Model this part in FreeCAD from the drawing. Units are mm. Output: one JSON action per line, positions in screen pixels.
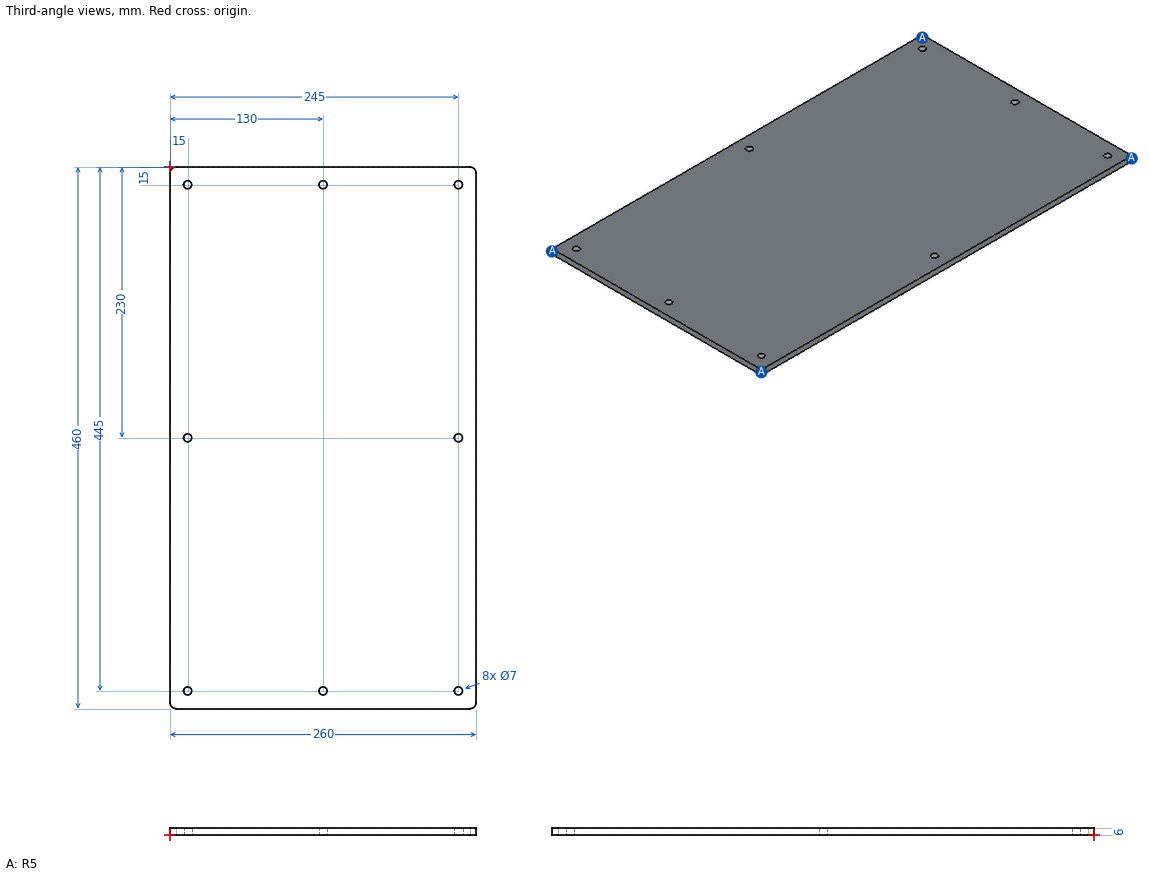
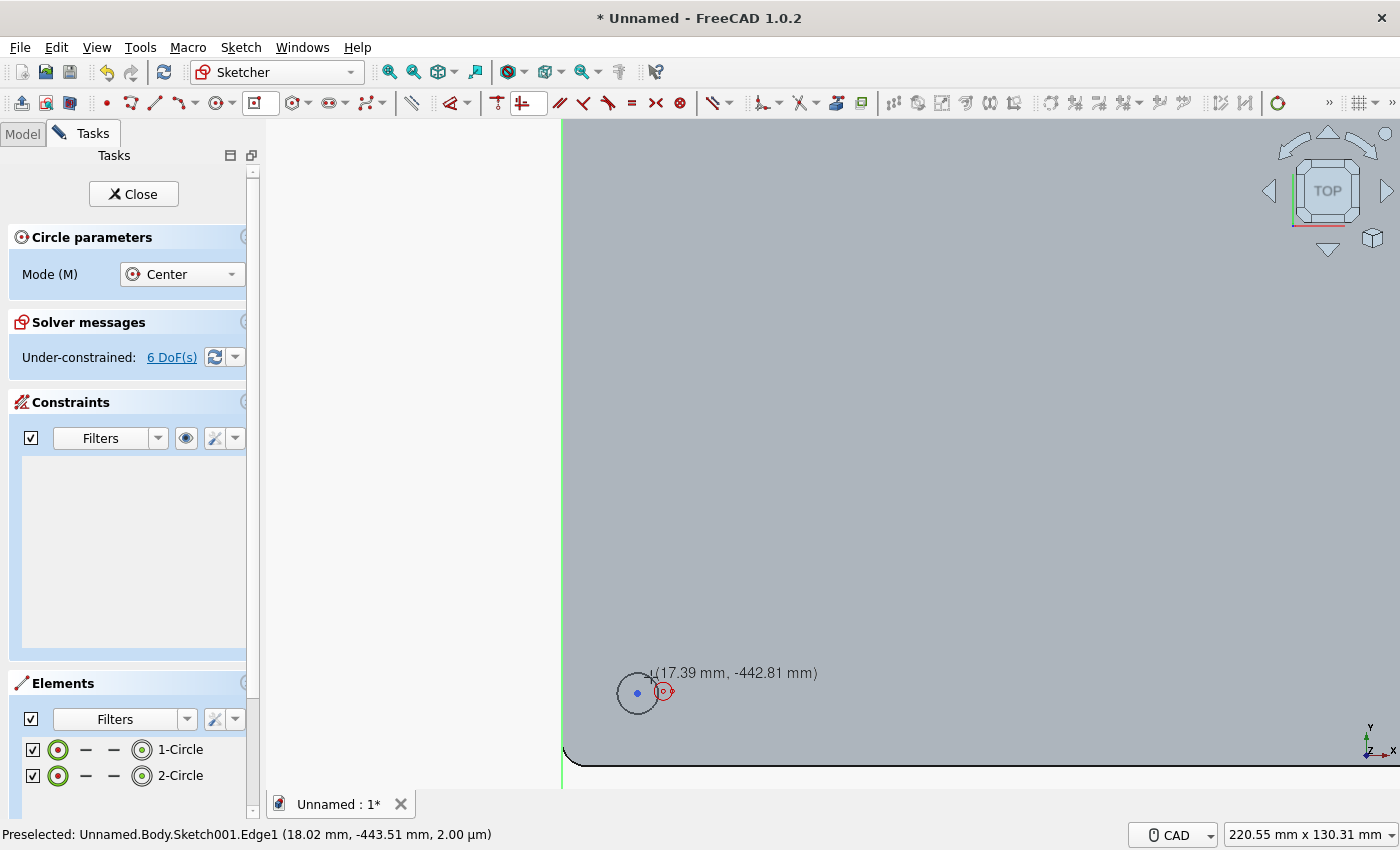
{"action": "scroll", "coordinate": [654, 682], "scroll_direction": "down", "scroll_amount": 8}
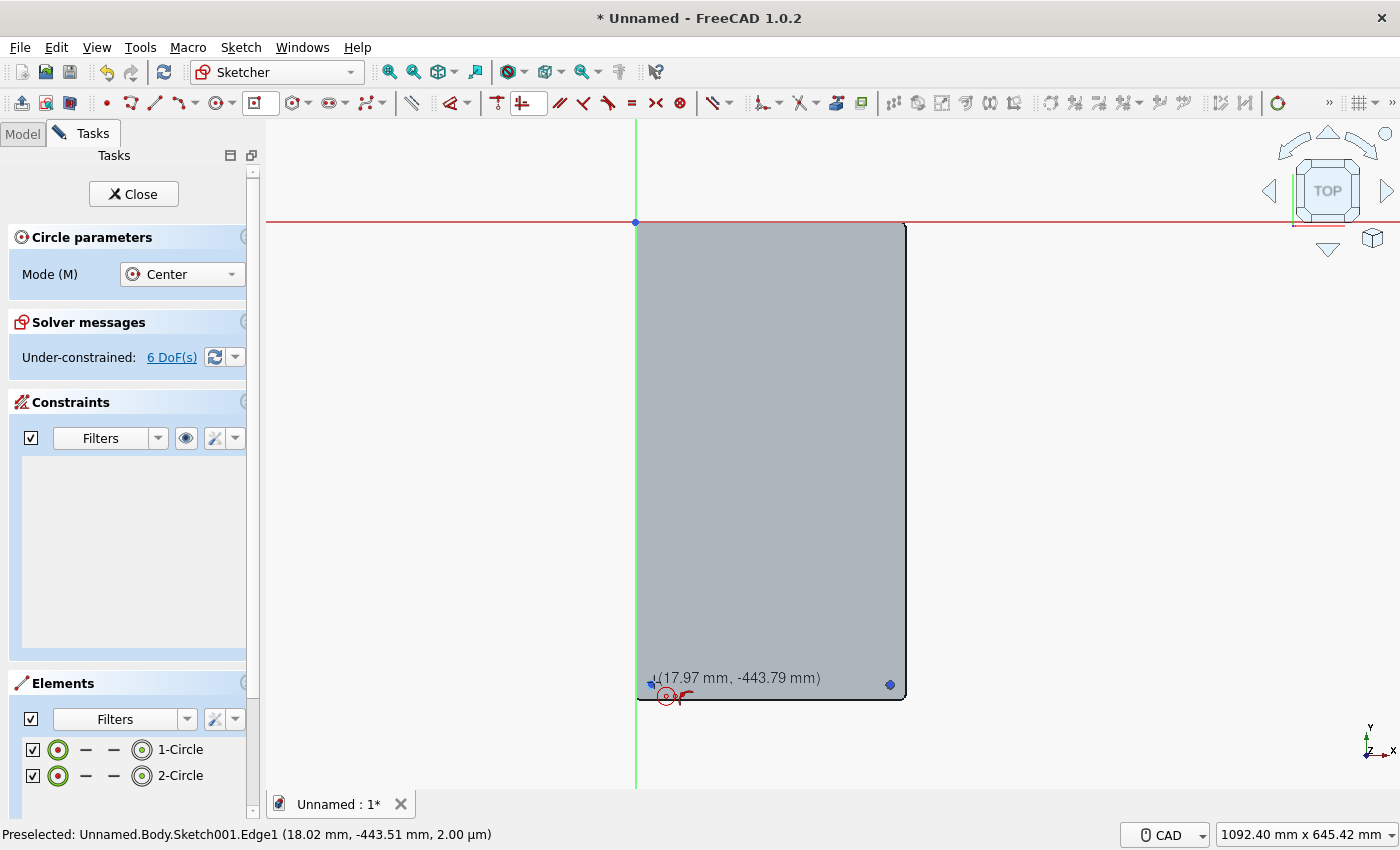
{"action": "scroll", "coordinate": [890, 238], "scroll_direction": "up", "scroll_amount": 10}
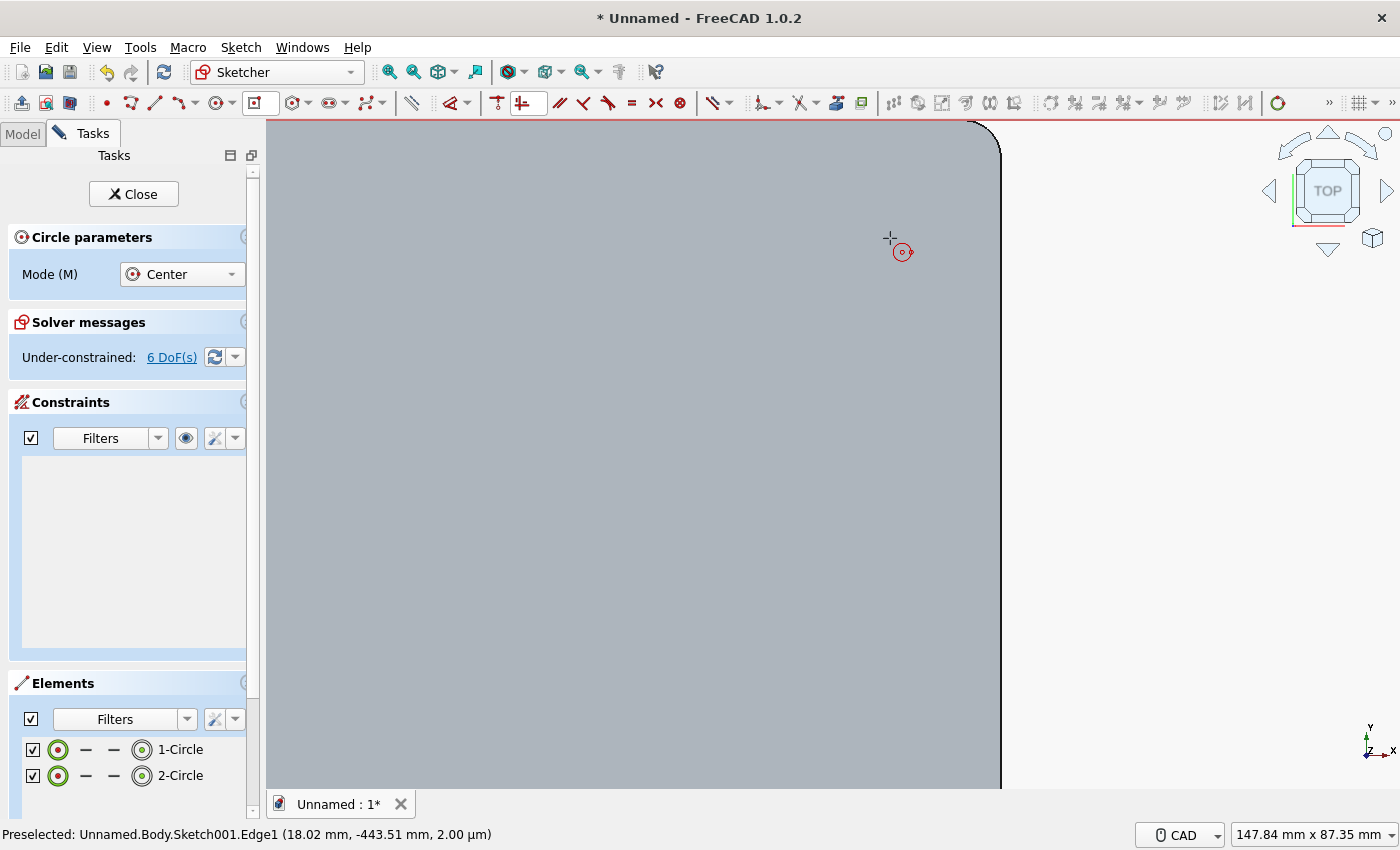
{"action": "scroll", "coordinate": [890, 237], "scroll_direction": "down", "scroll_amount": 10}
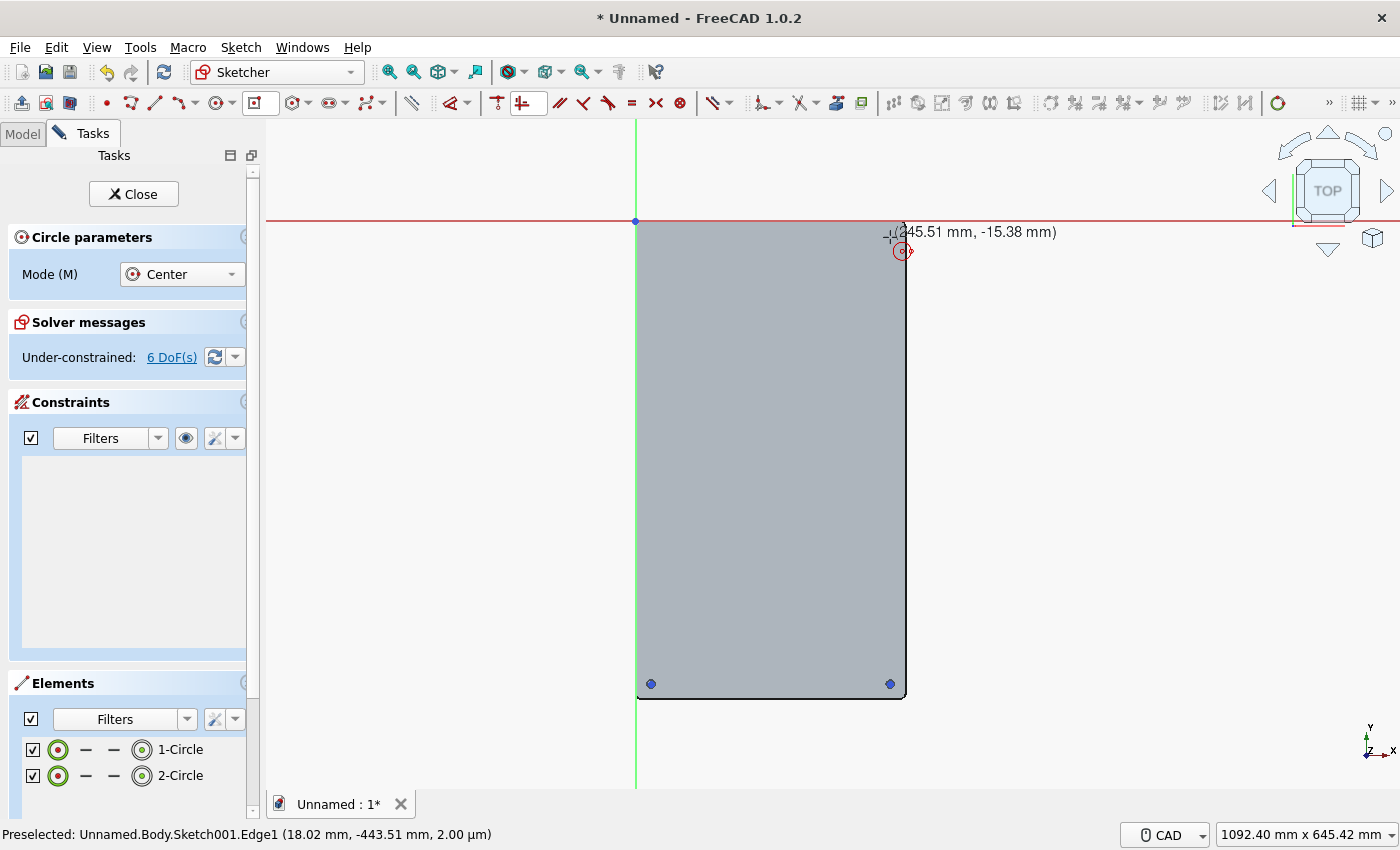
{"action": "left_click", "coordinate": [890, 237]}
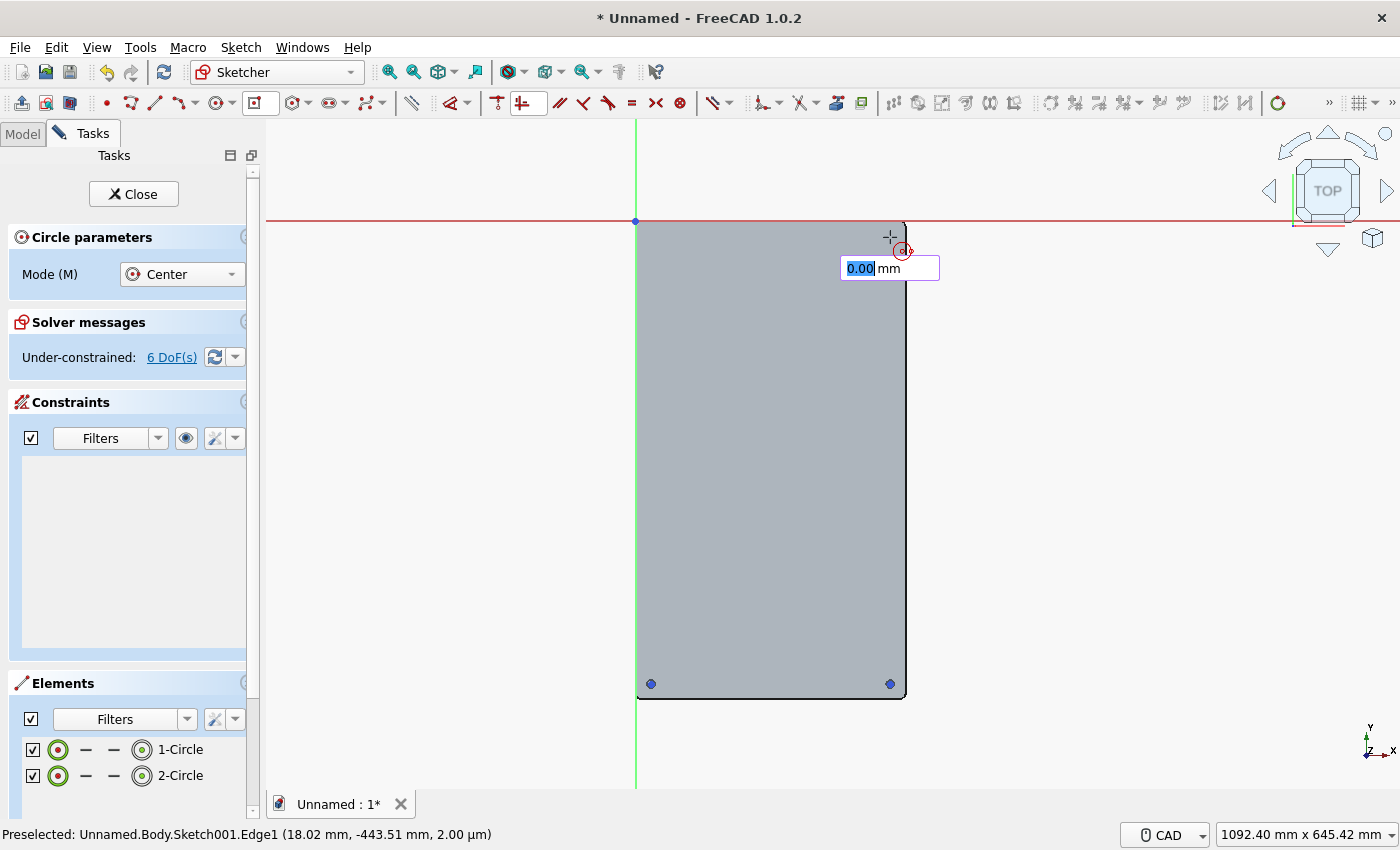
{"action": "scroll", "coordinate": [893, 239], "scroll_direction": "up", "scroll_amount": 8}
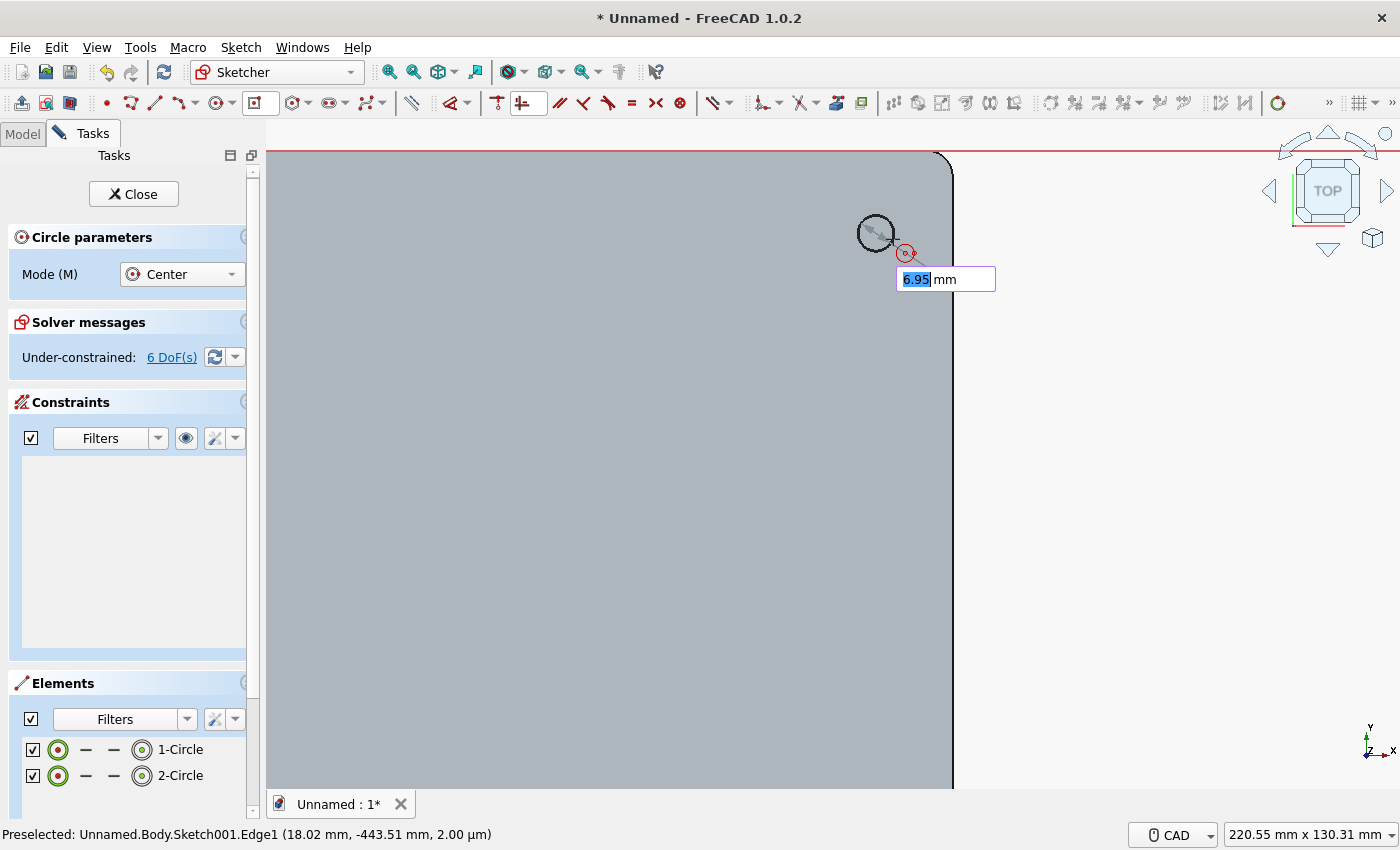
{"action": "left_click", "coordinate": [888, 241]}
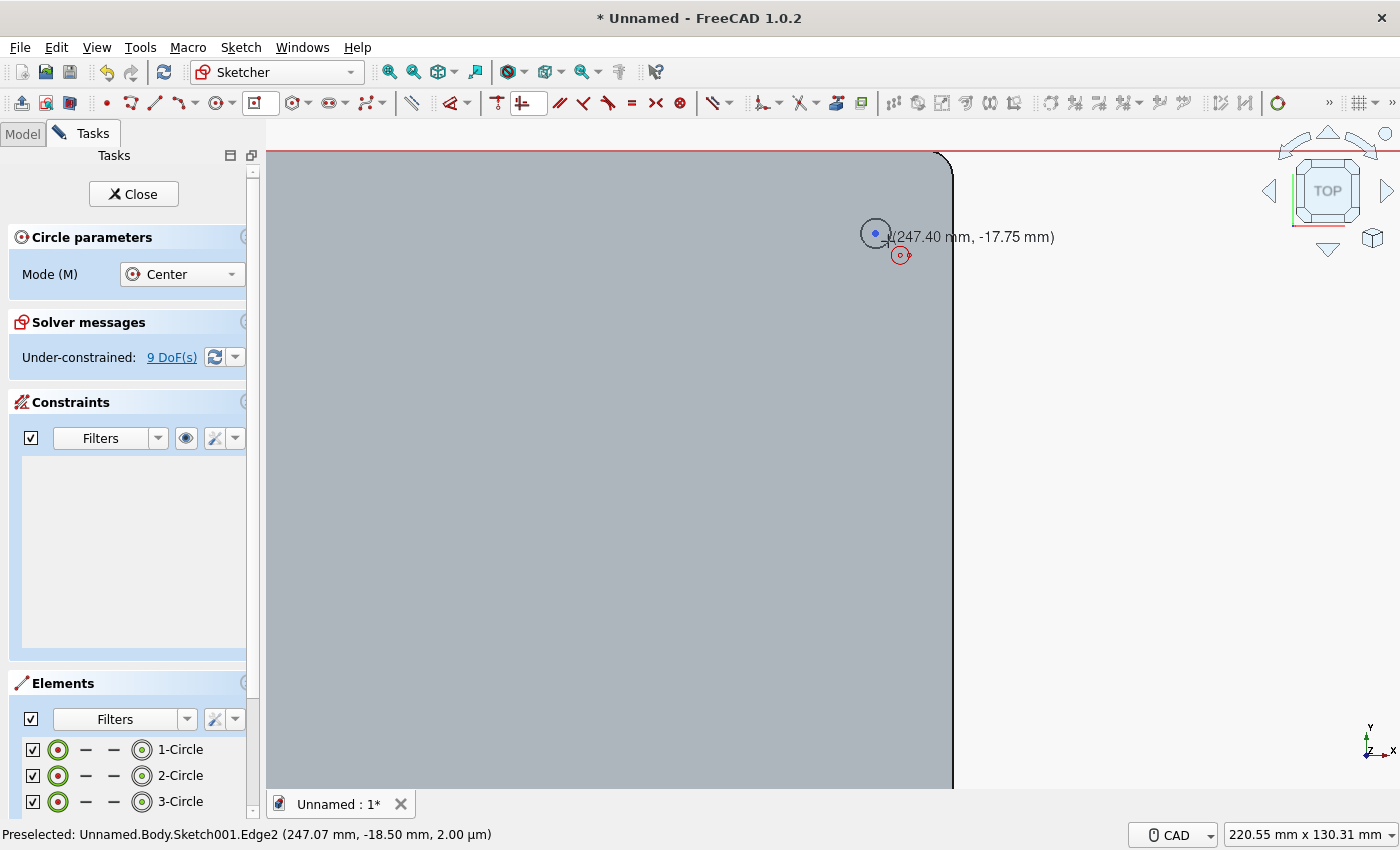
{"action": "scroll", "coordinate": [893, 239], "scroll_direction": "down", "scroll_amount": 8}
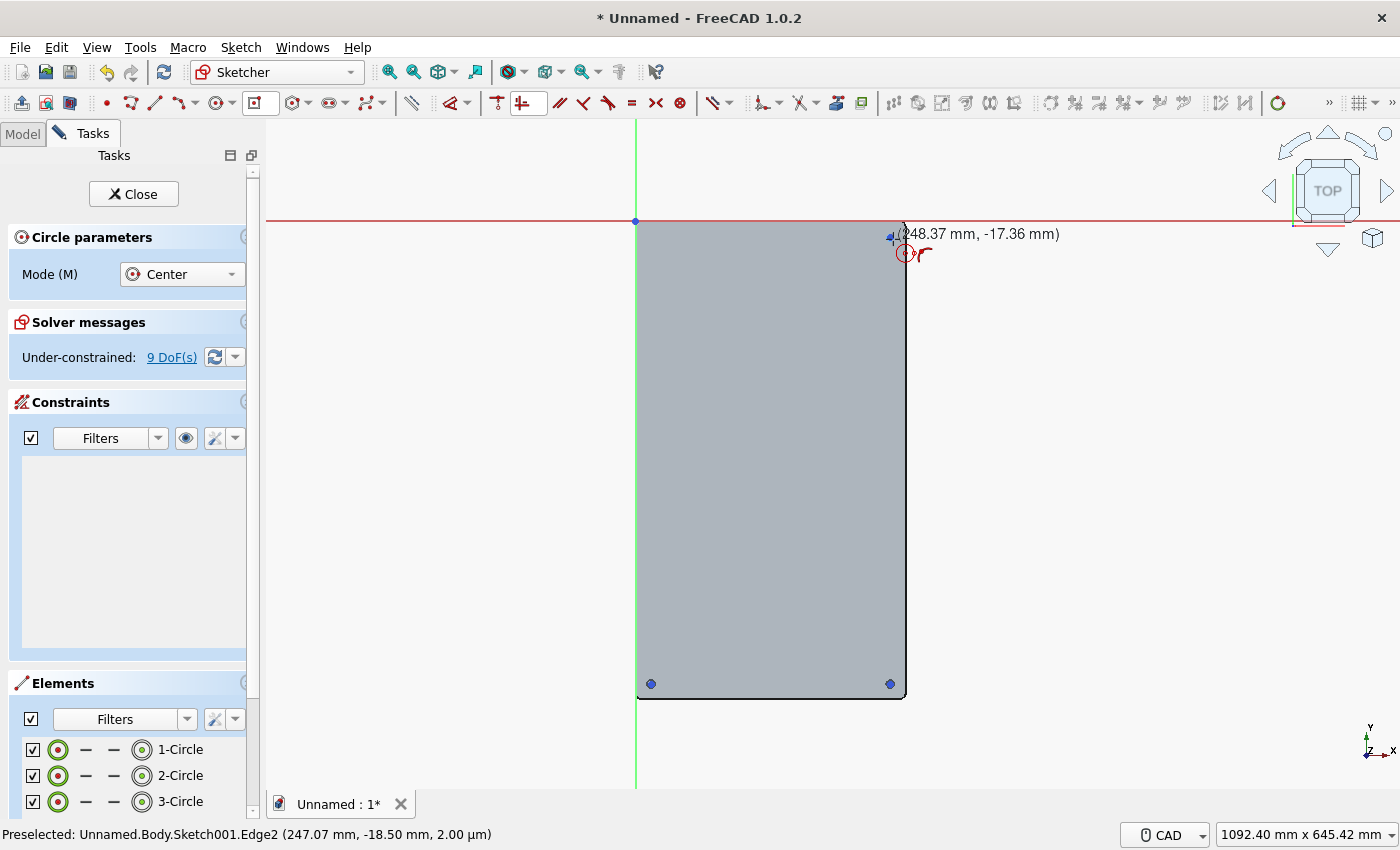
{"action": "scroll", "coordinate": [651, 237], "scroll_direction": "up", "scroll_amount": 10}